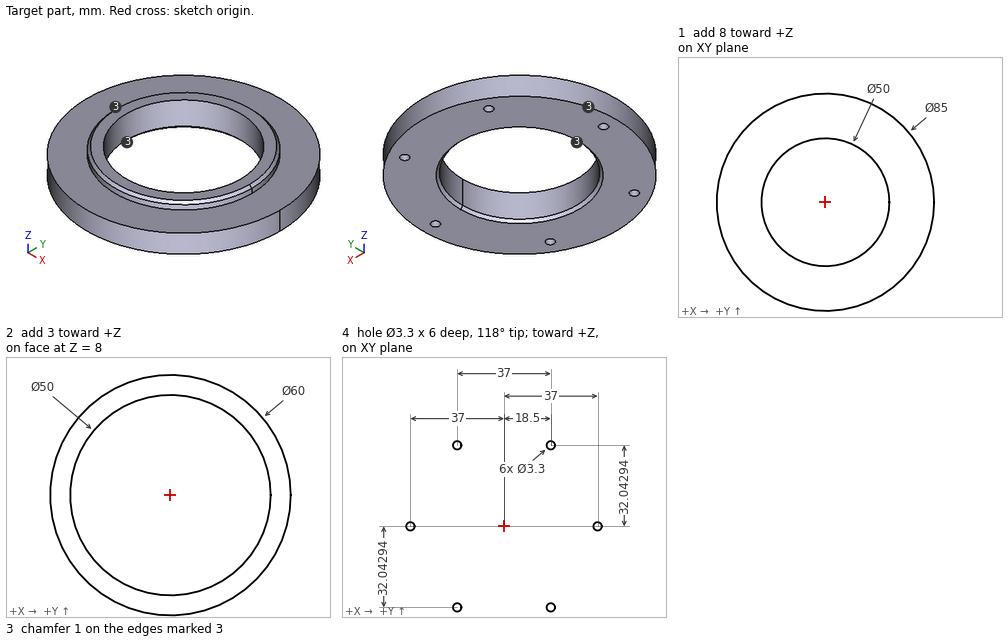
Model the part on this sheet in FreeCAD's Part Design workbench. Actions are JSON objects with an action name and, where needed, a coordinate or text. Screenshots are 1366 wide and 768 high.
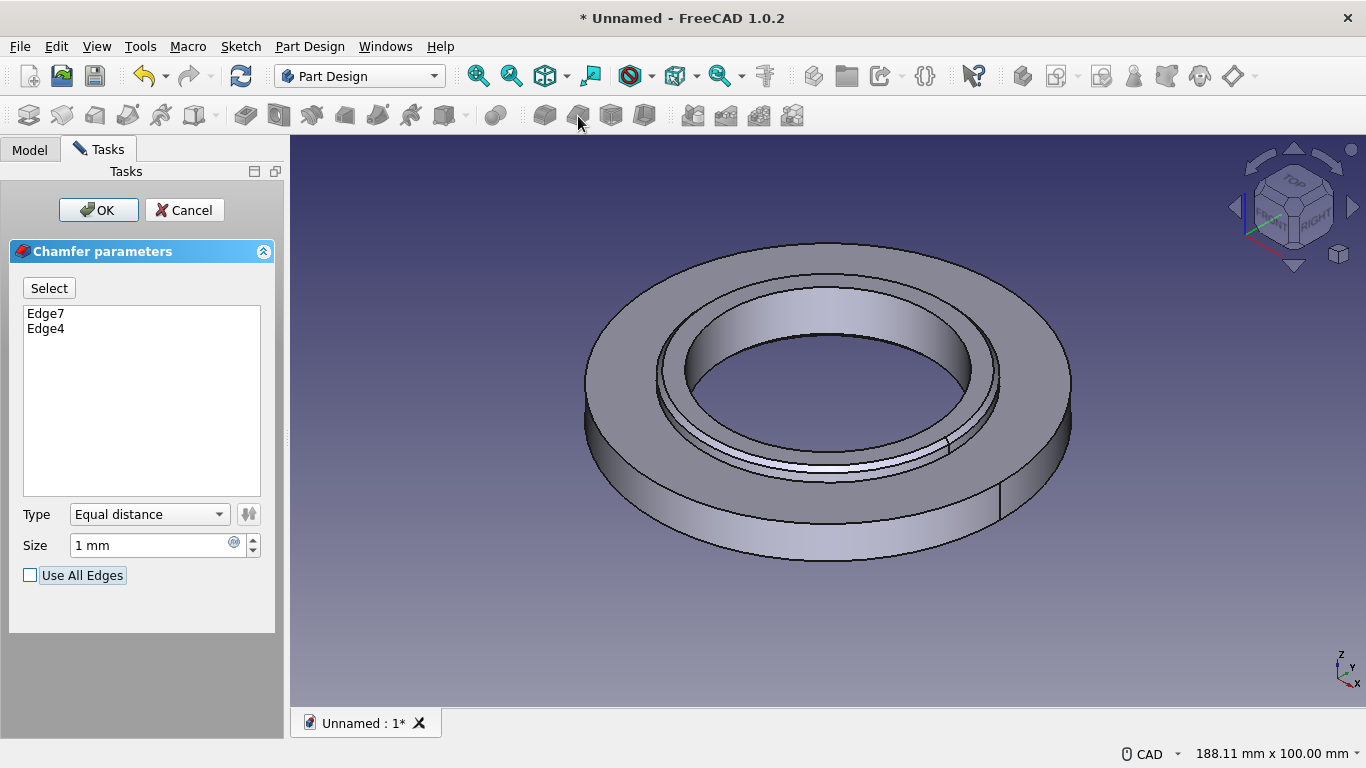
{"action": "left_click", "coordinate": [99, 210]}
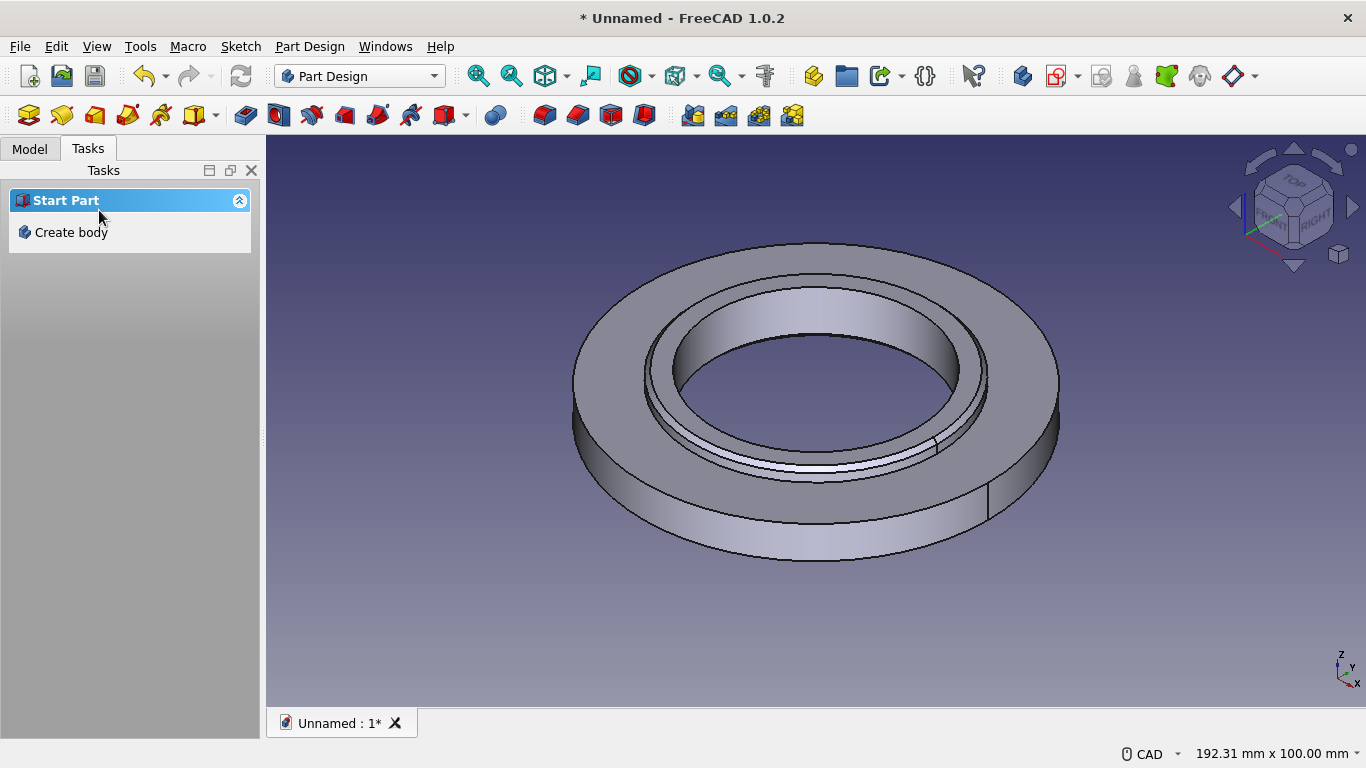
{"action": "left_click", "coordinate": [1056, 76]}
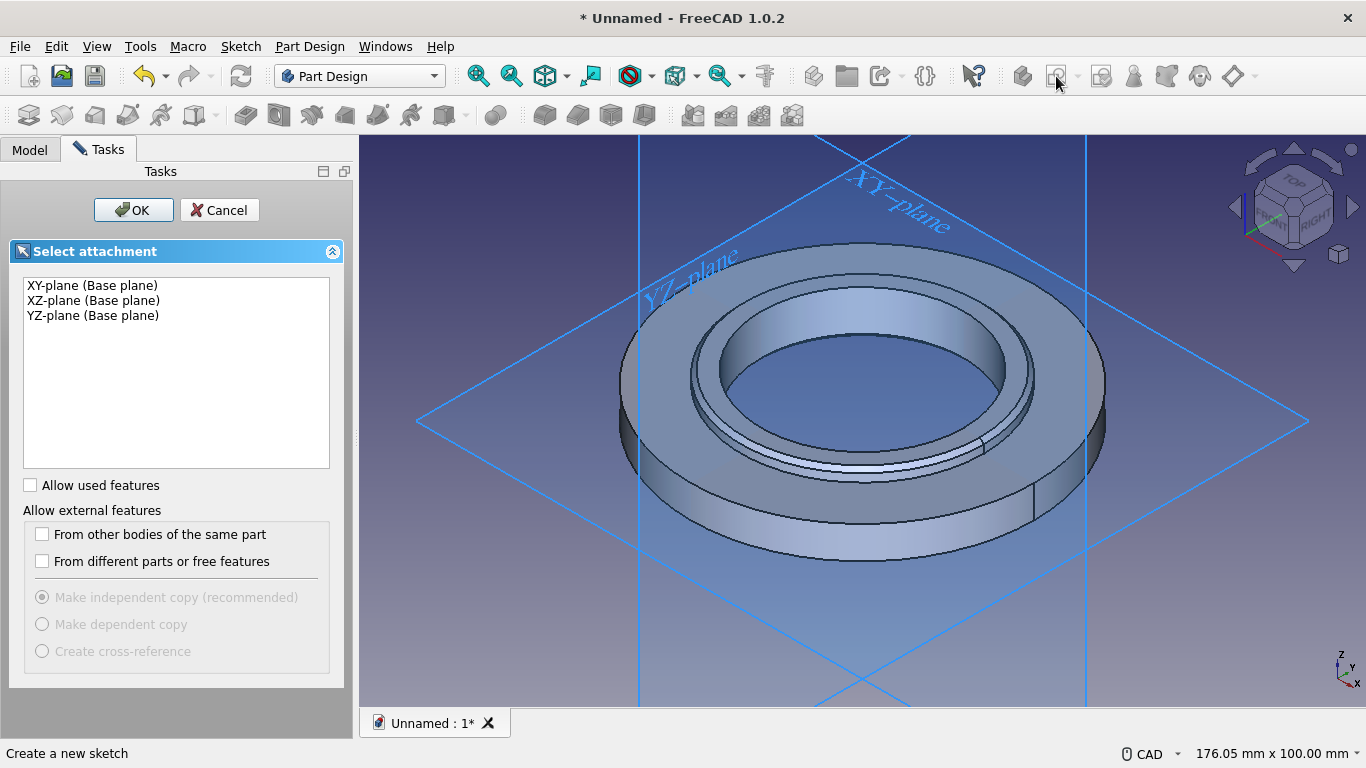
{"action": "left_click", "coordinate": [84, 286]}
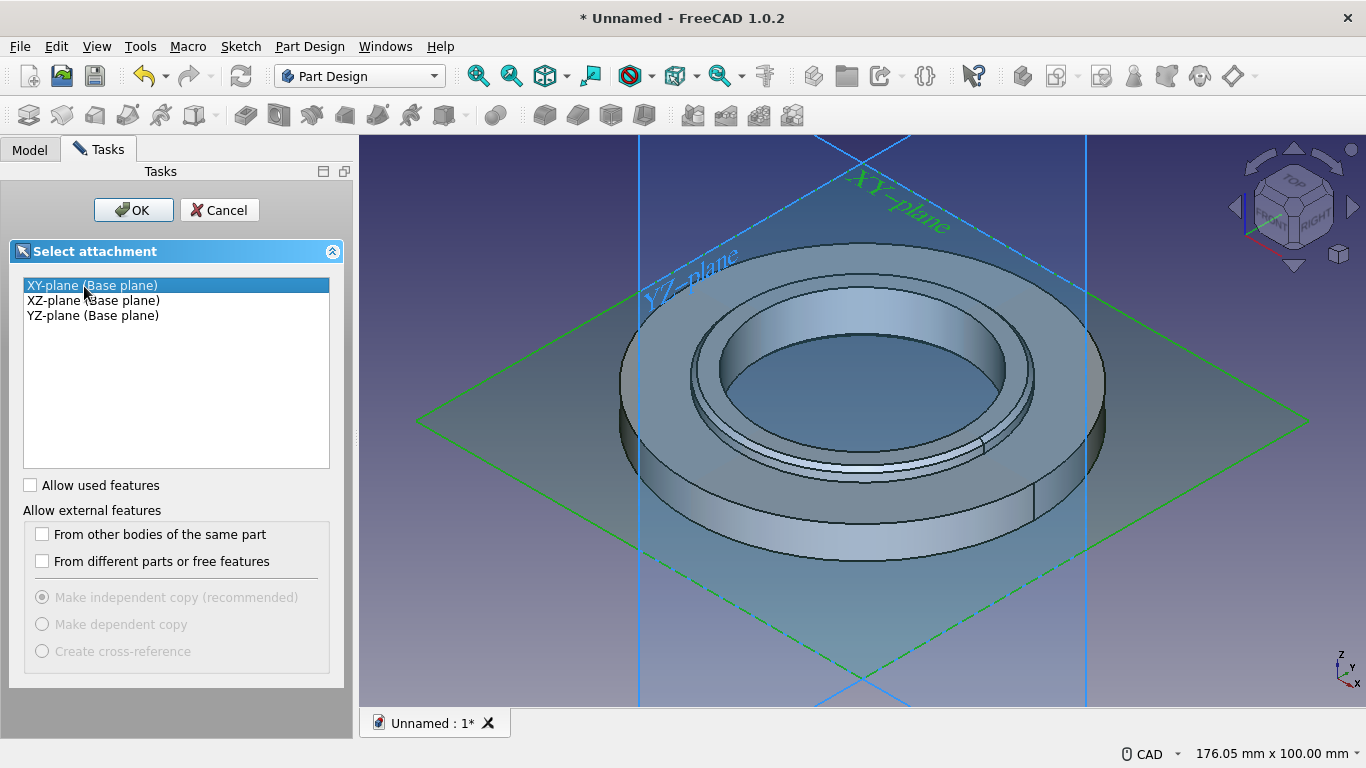
{"action": "left_click", "coordinate": [134, 210]}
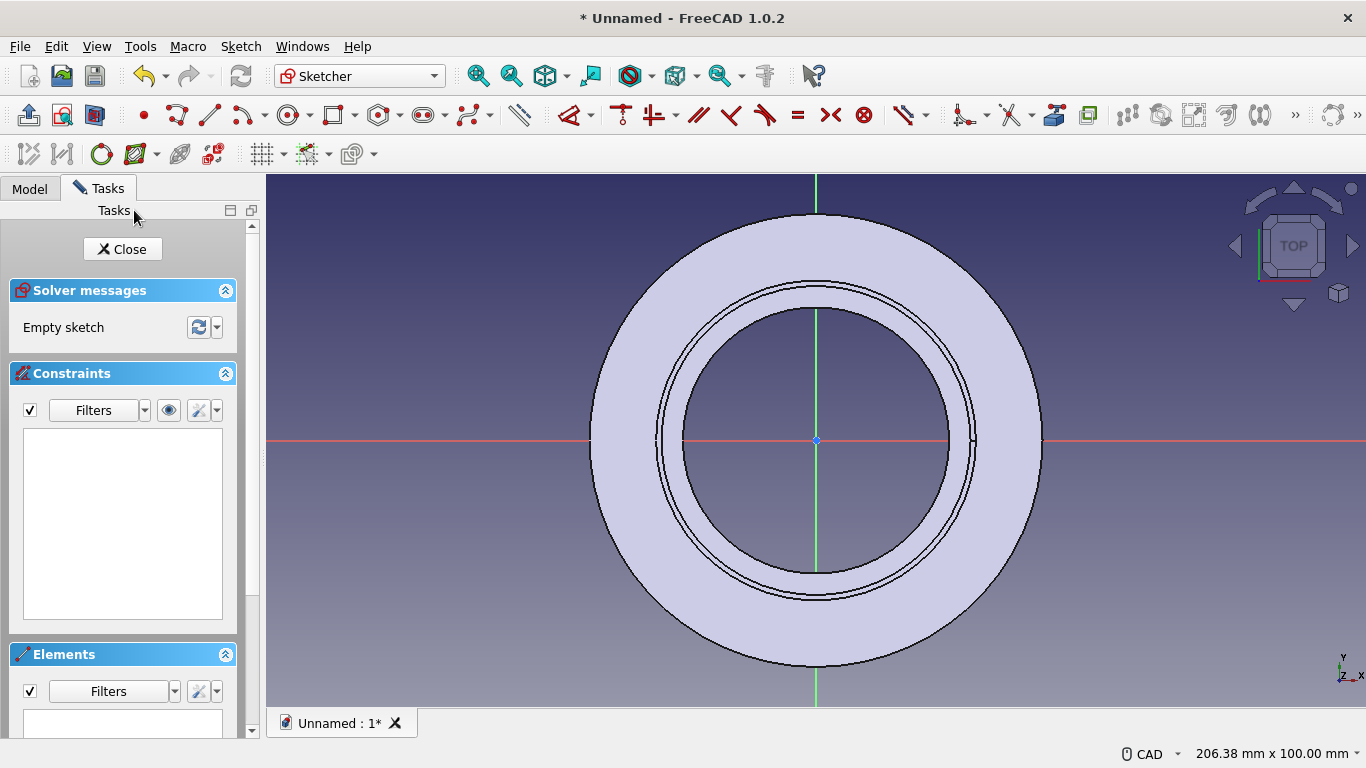
{"action": "left_click", "coordinate": [95, 116]}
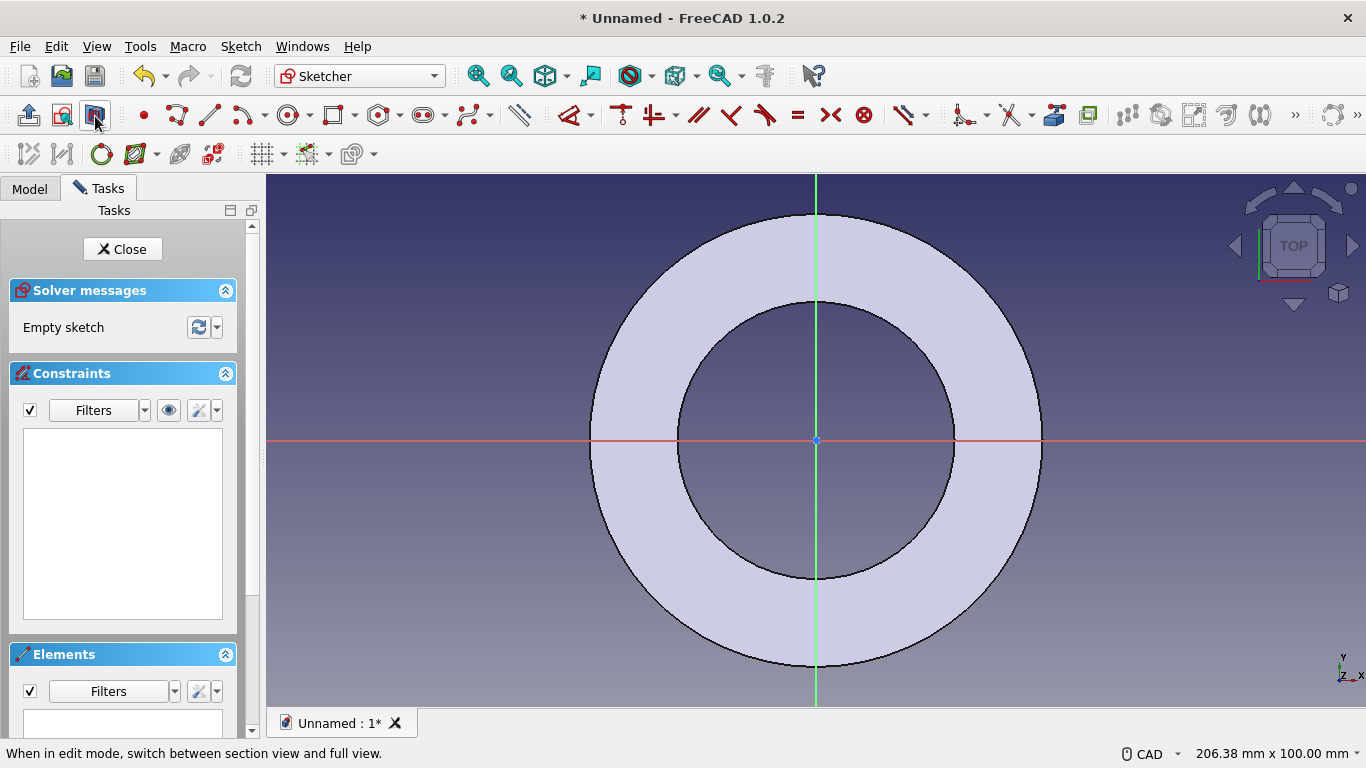
{"action": "left_click", "coordinate": [288, 116]}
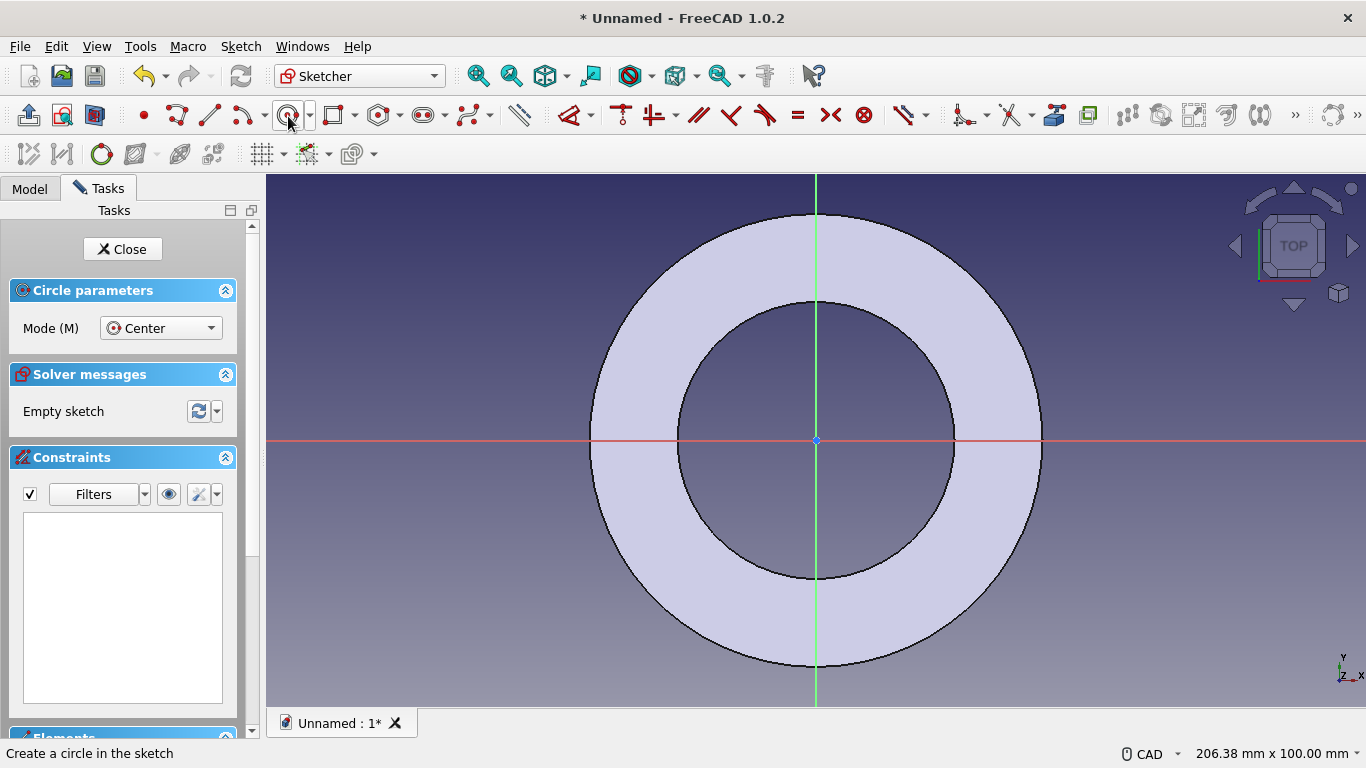
{"action": "scroll", "coordinate": [915, 270], "scroll_direction": "up", "scroll_amount": 5}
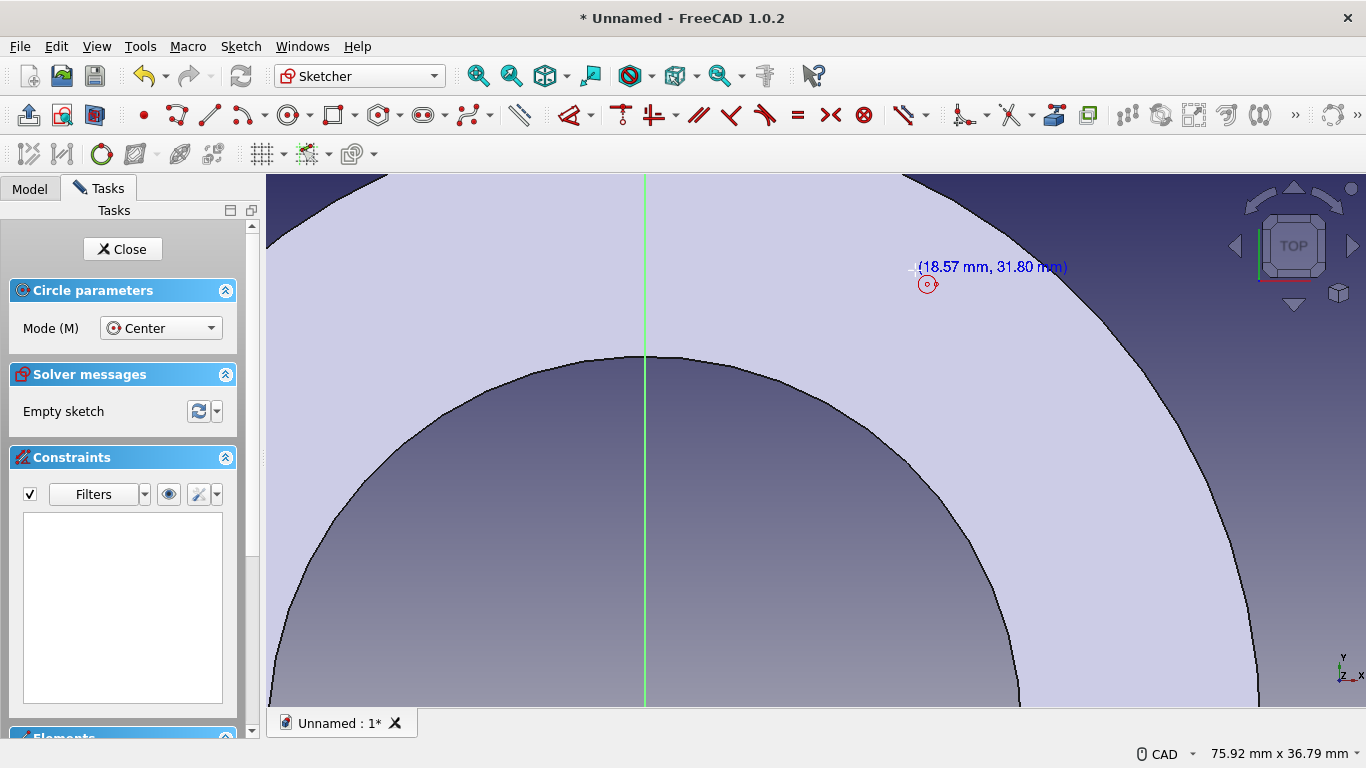
{"action": "left_click", "coordinate": [913, 269]}
{"action": "mouse_move", "coordinate": [930, 252]}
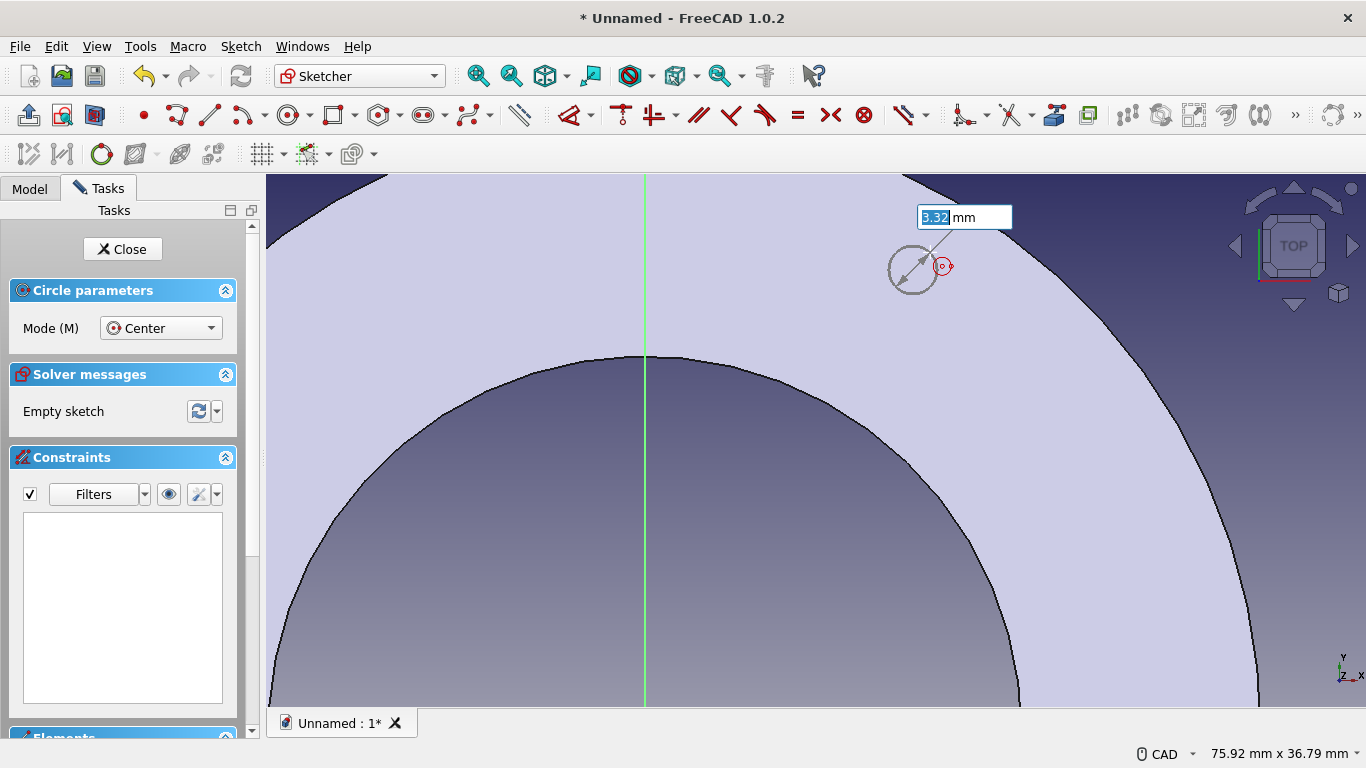
{"action": "type", "text": "3.3"}
{"action": "key", "text": "Return"}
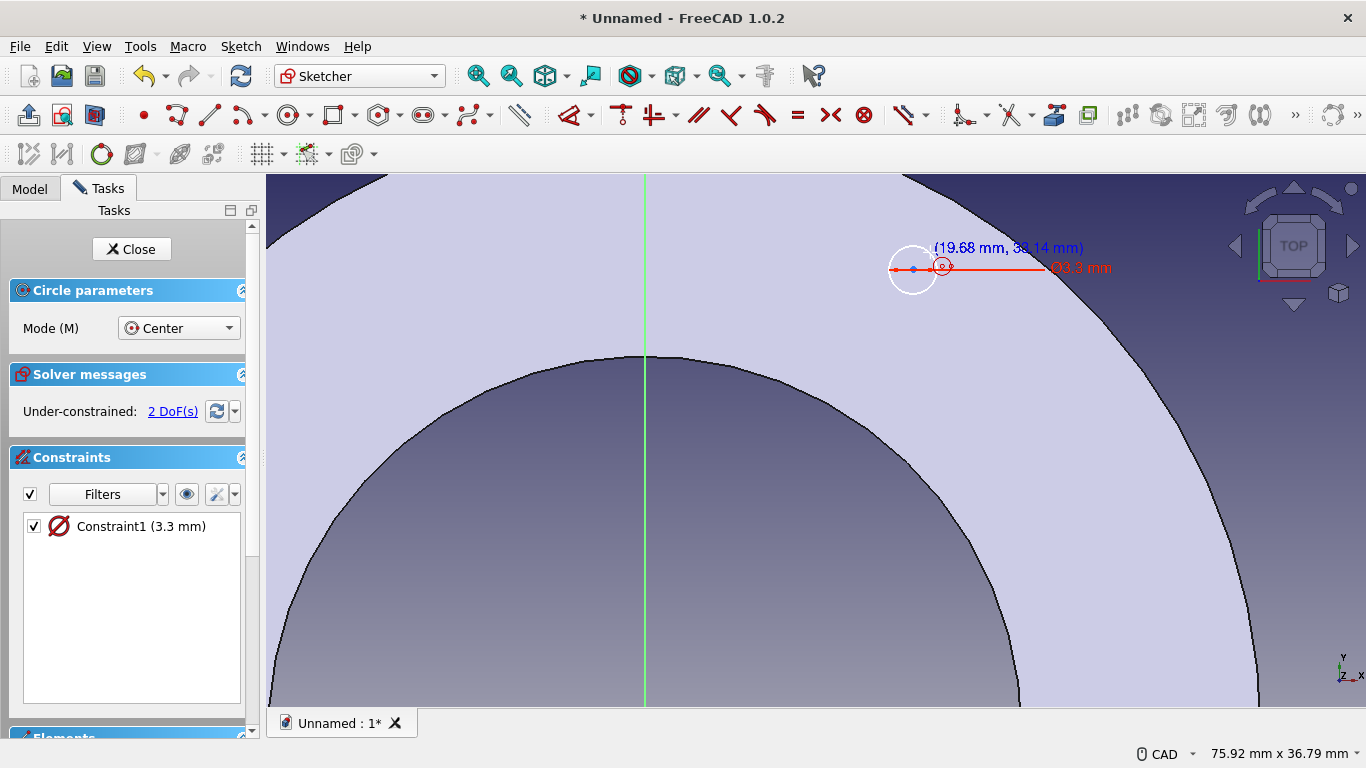
{"action": "left_click", "coordinate": [377, 269]}
{"action": "mouse_move", "coordinate": [394, 252]}